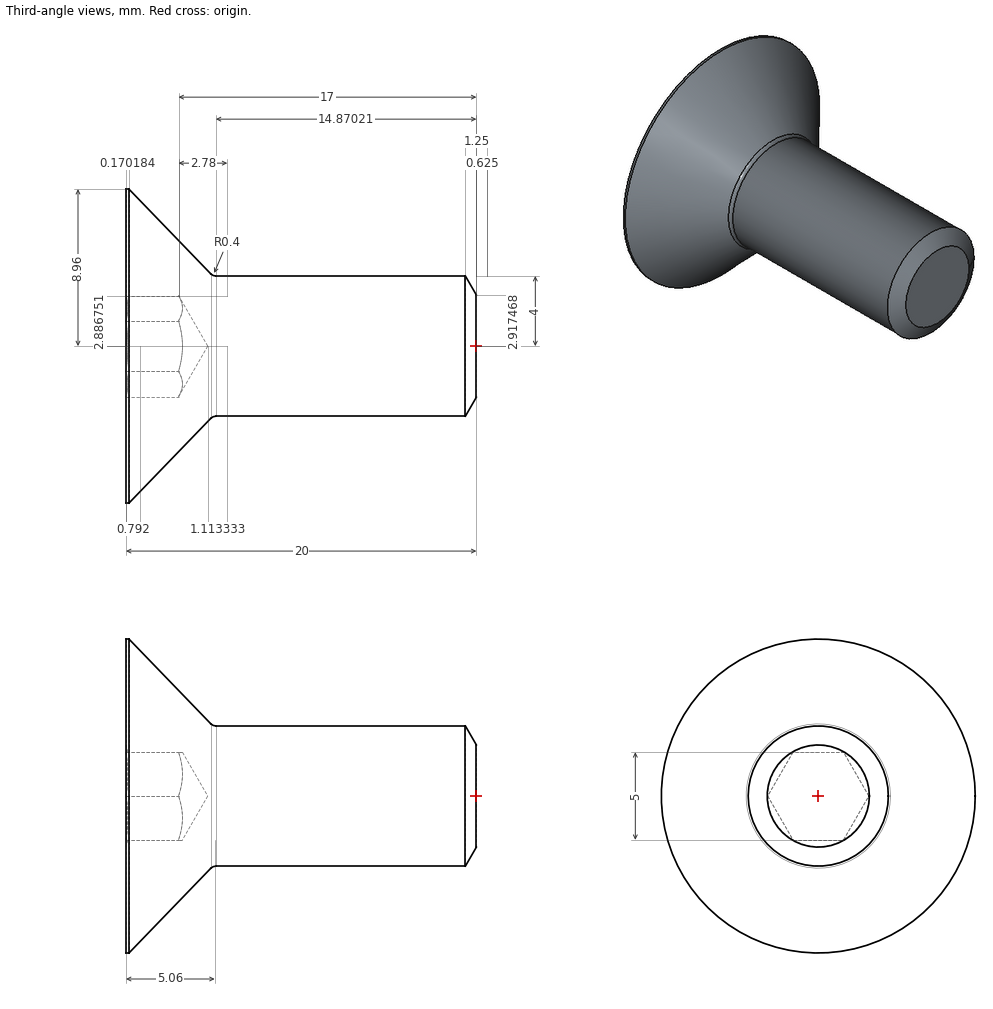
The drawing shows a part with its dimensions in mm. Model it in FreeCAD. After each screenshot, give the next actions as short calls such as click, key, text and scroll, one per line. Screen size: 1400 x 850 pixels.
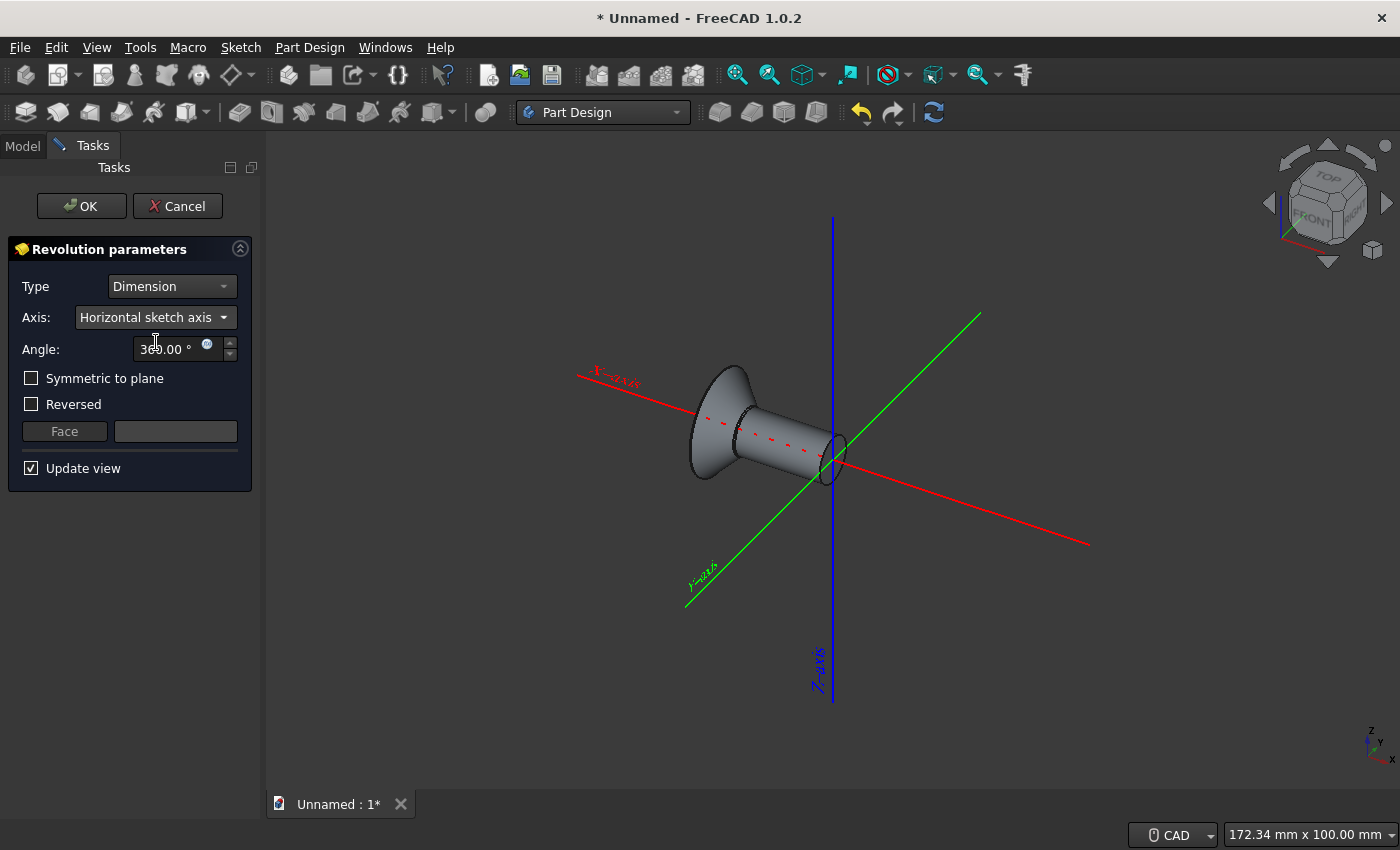
click(82, 206)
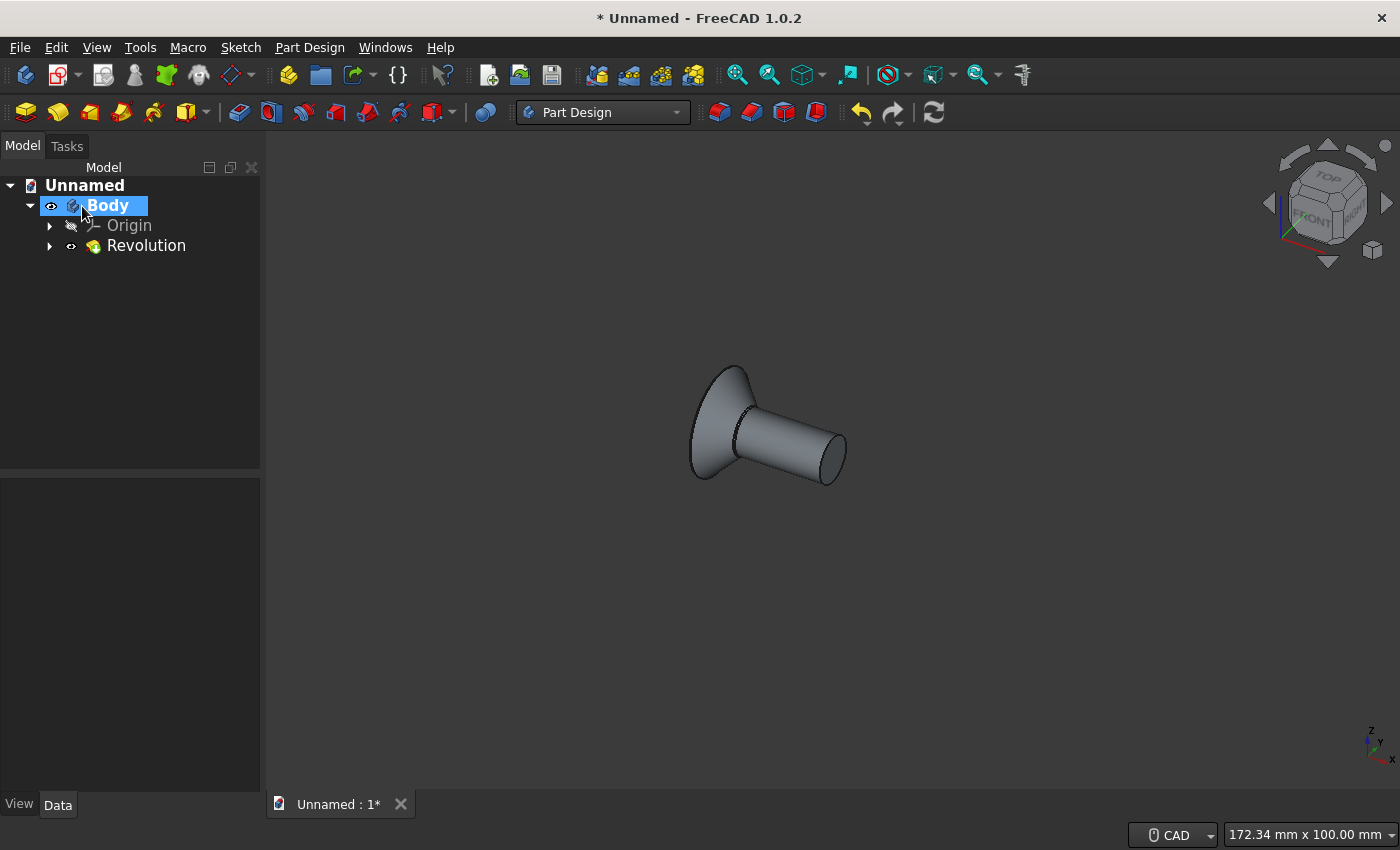
click(738, 76)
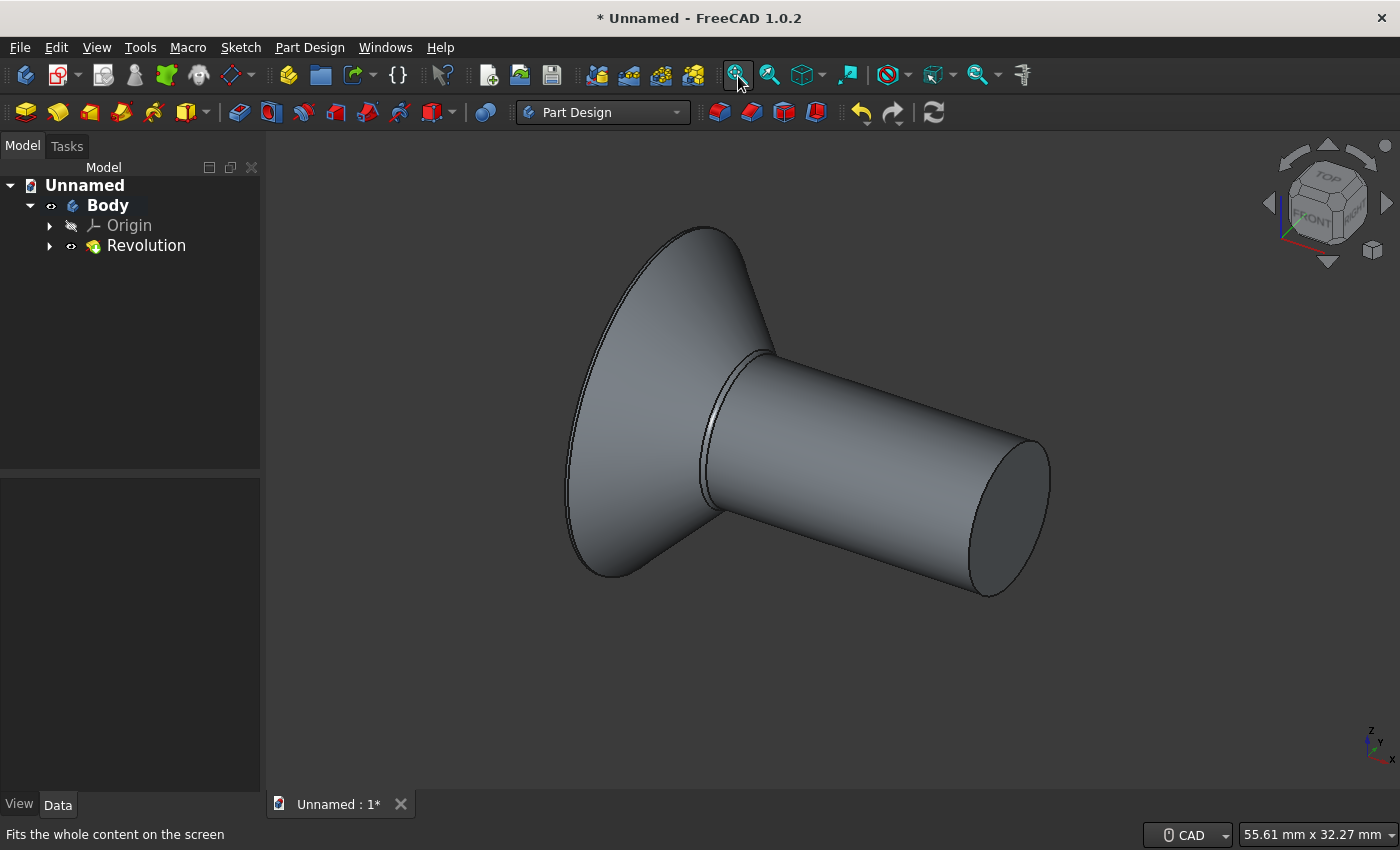
key(6)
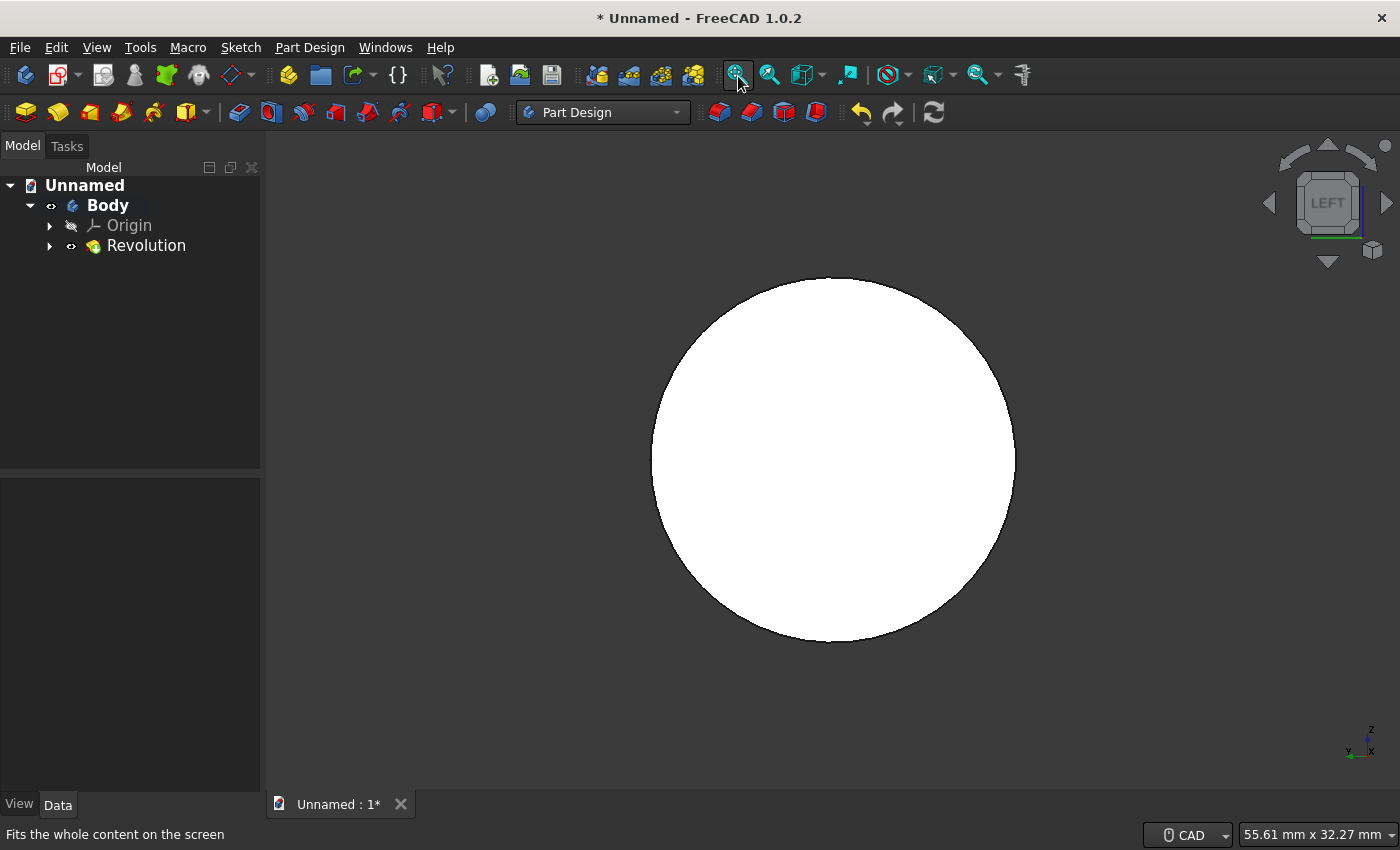
click(833, 459)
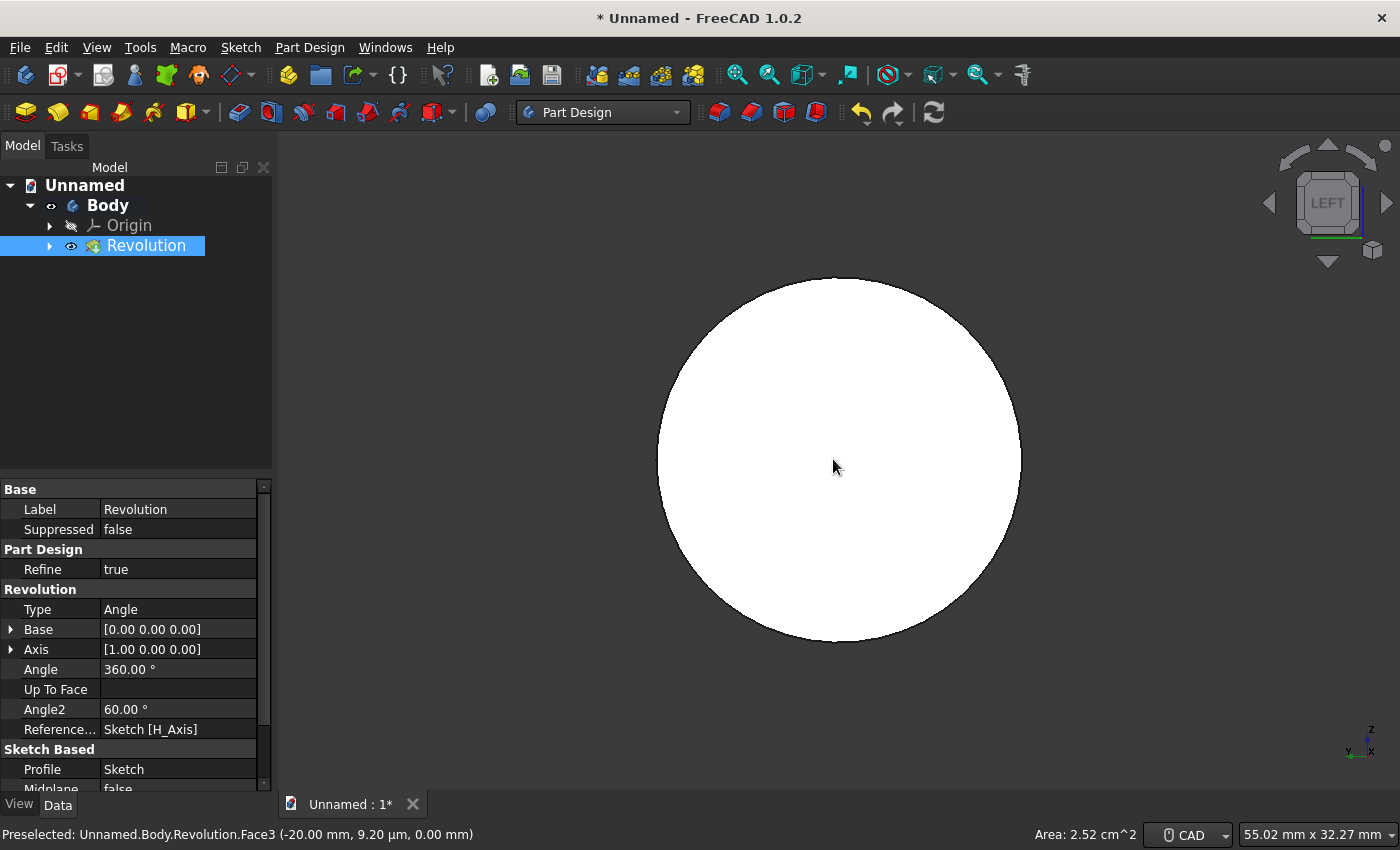
click(58, 76)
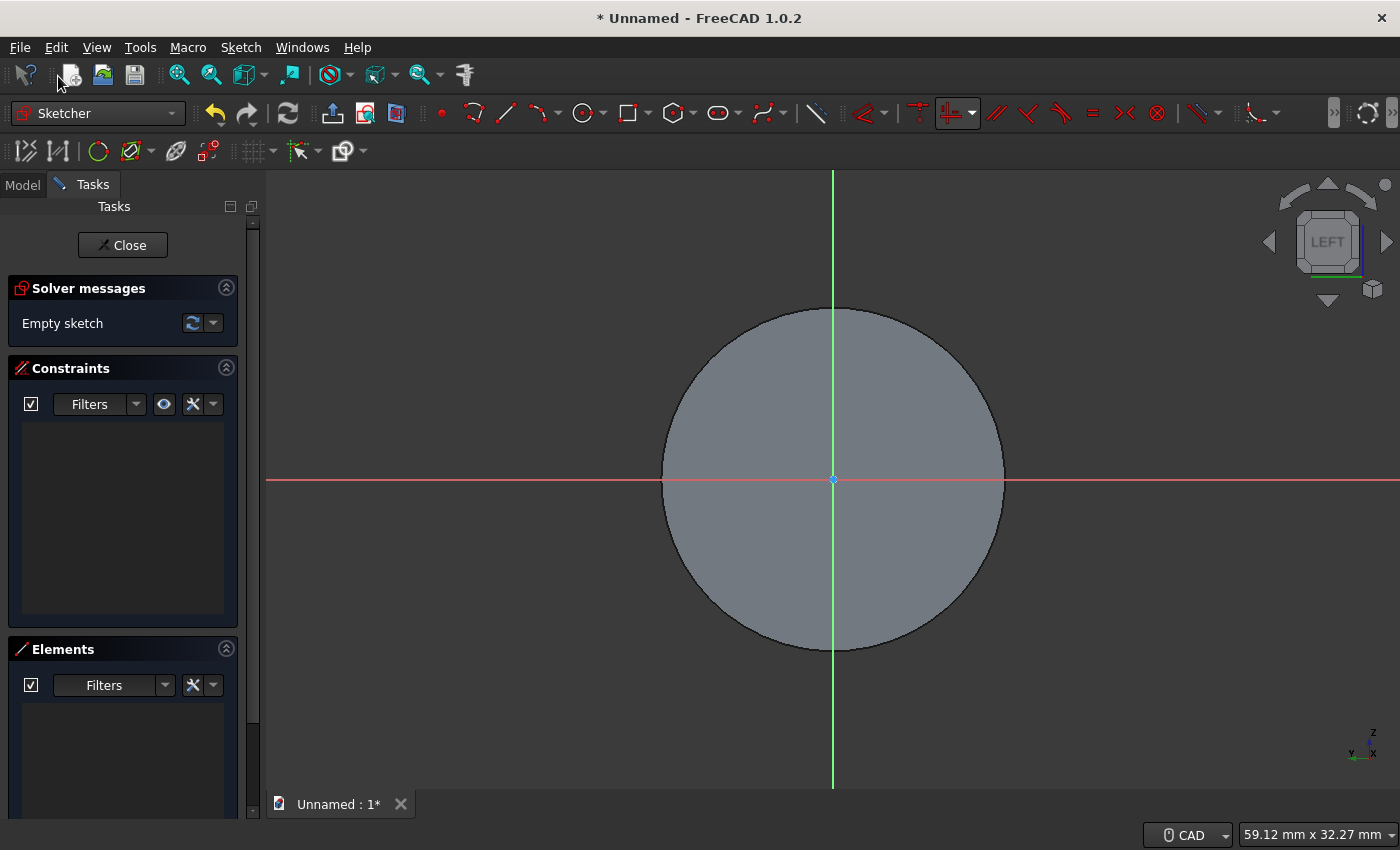
scroll(856, 480, up, 7)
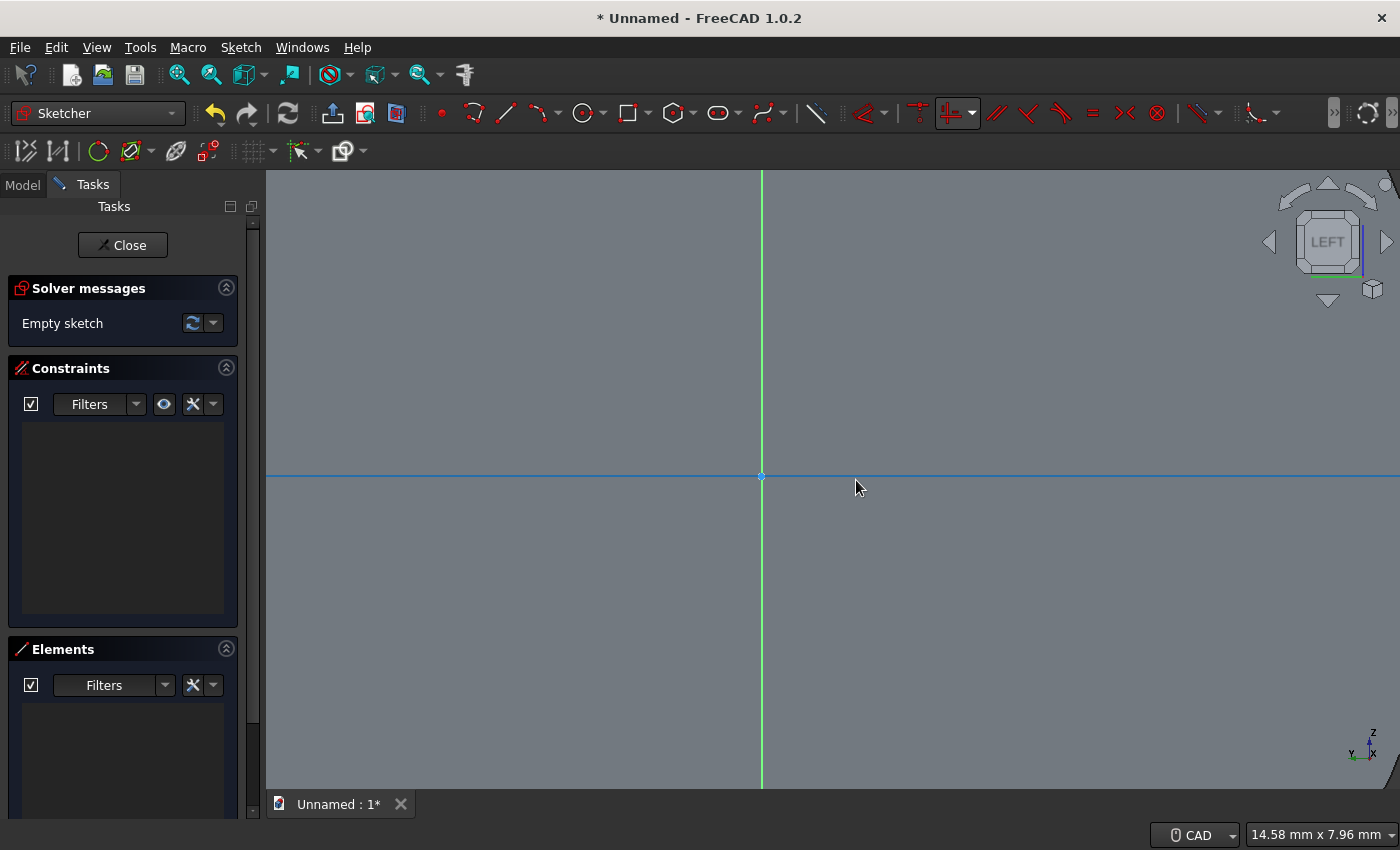
click(674, 114)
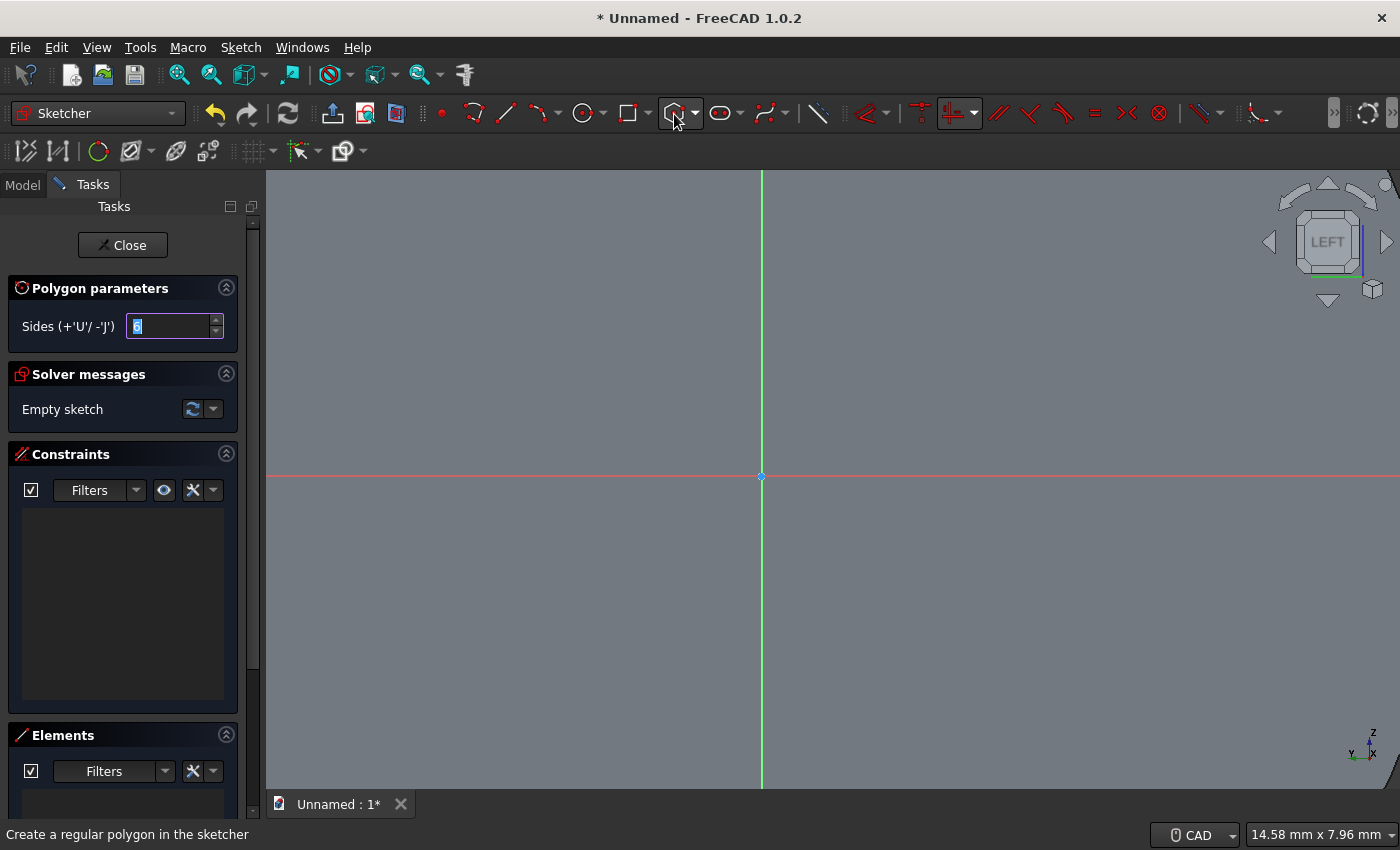
click(762, 476)